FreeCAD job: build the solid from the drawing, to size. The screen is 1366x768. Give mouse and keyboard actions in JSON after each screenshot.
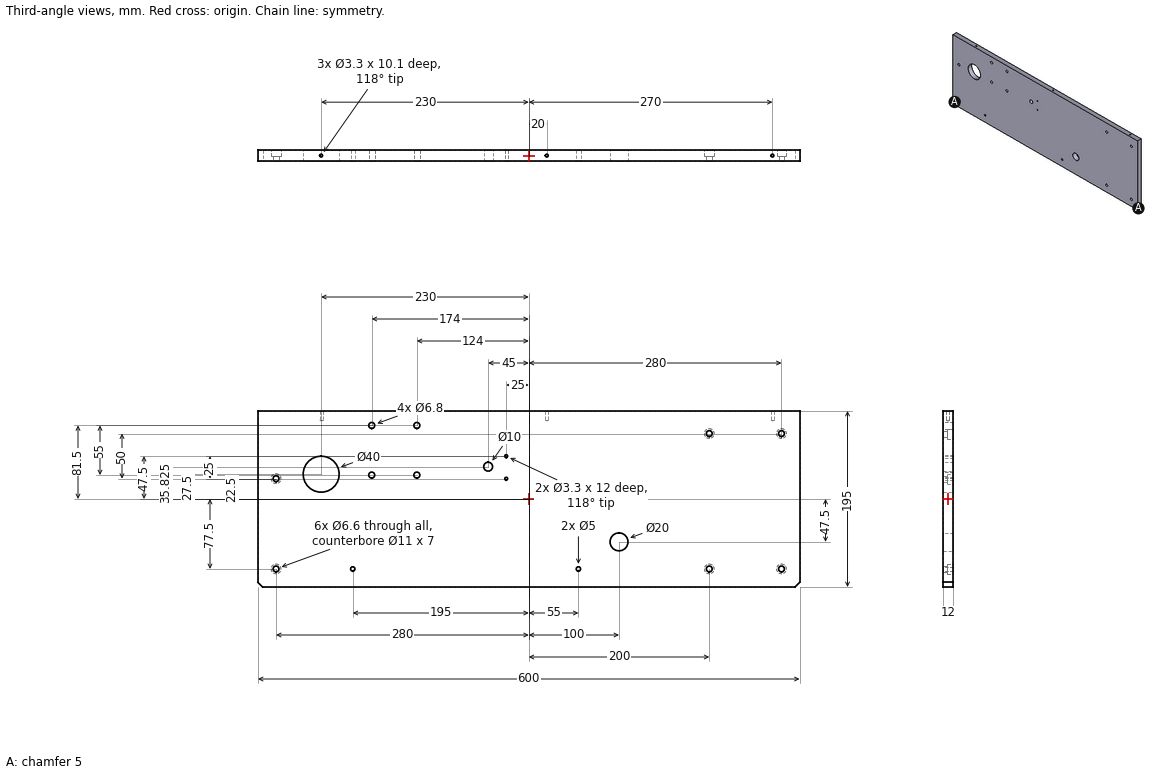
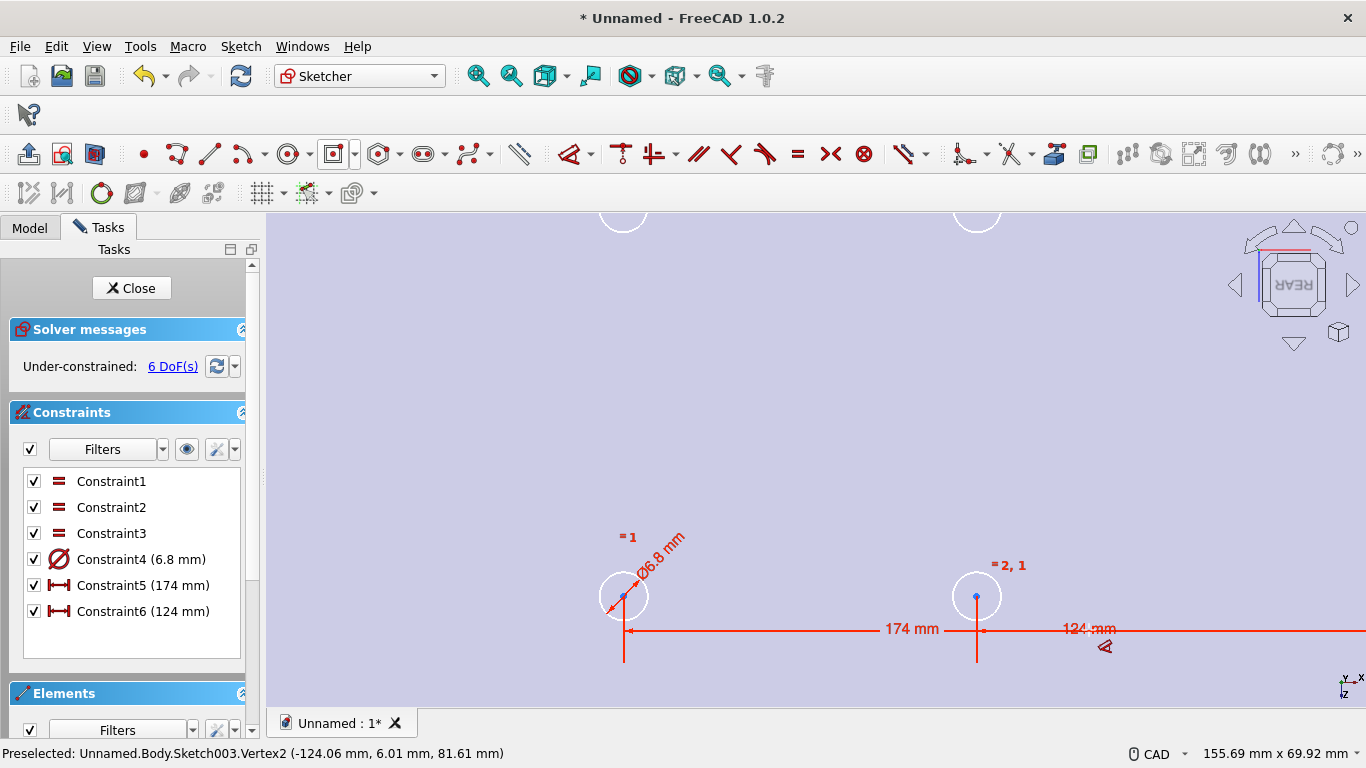
{"action": "scroll", "coordinate": [640, 579], "scroll_direction": "down", "scroll_amount": 2}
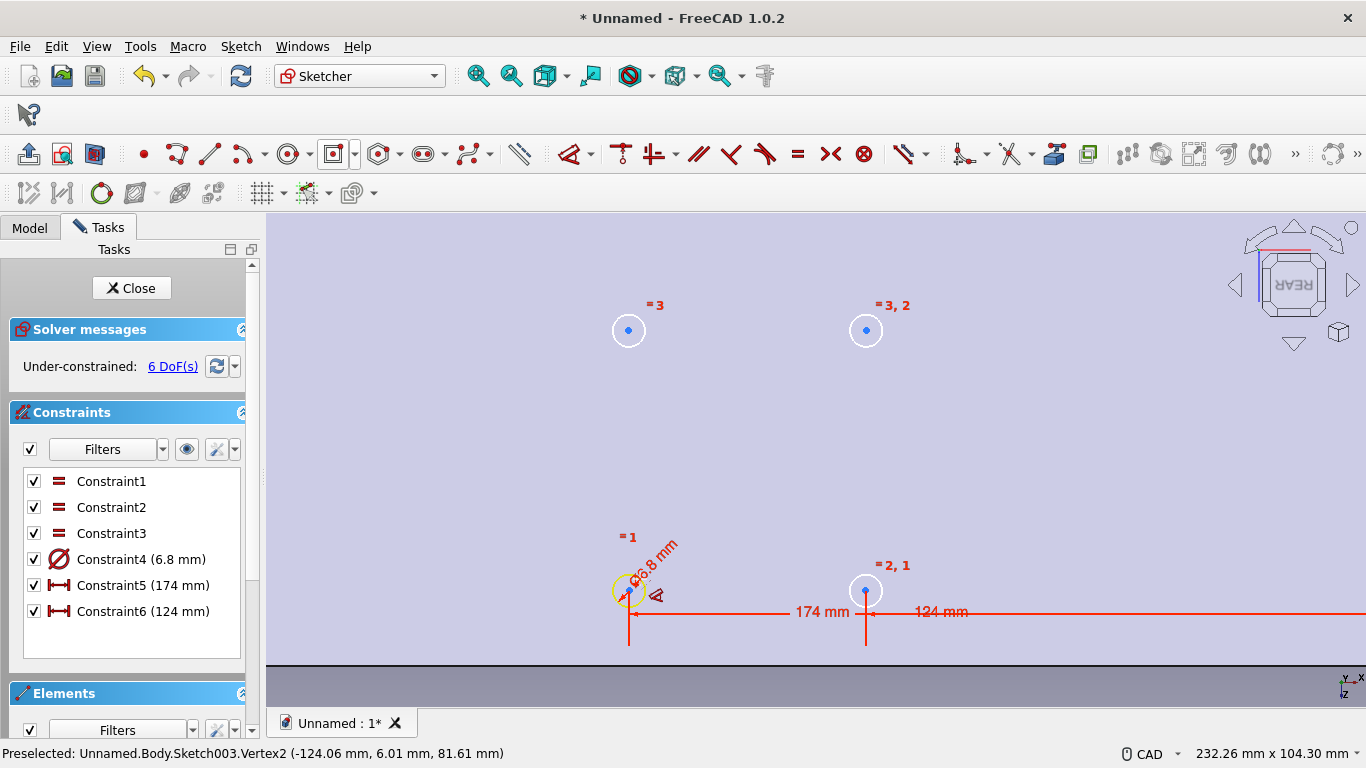
{"action": "left_click", "coordinate": [866, 331]}
{"action": "left_click", "coordinate": [1034, 365]}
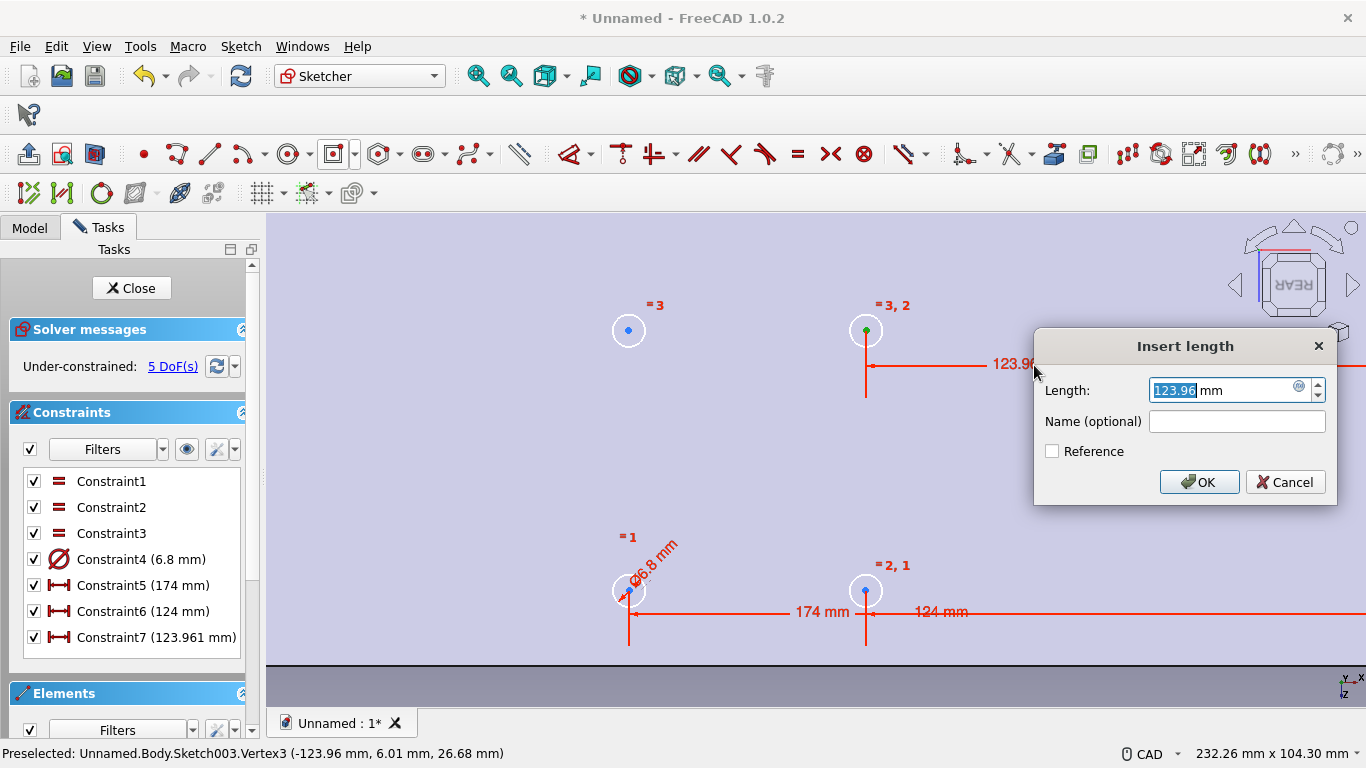
{"action": "type", "text": "124"}
{"action": "key", "text": "Return"}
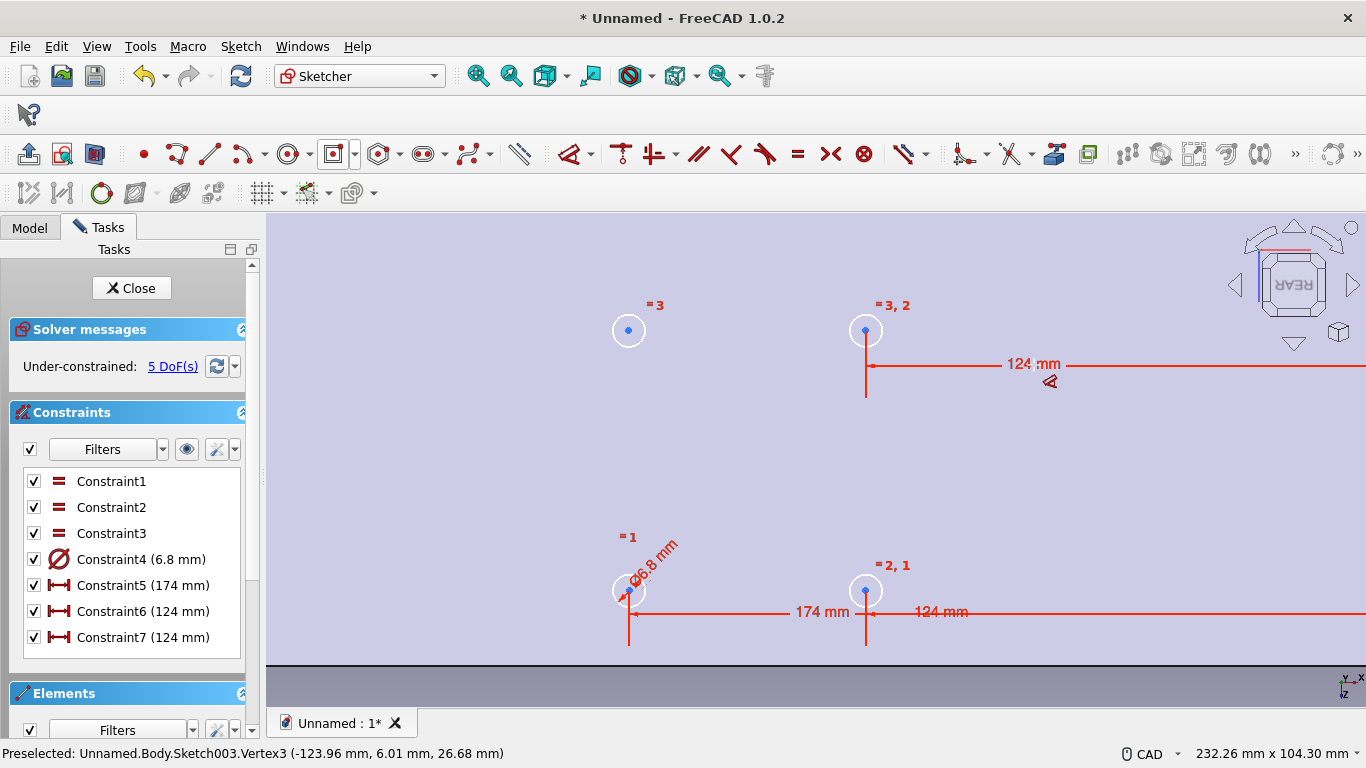
{"action": "left_click", "coordinate": [629, 331]}
{"action": "left_click", "coordinate": [915, 365]}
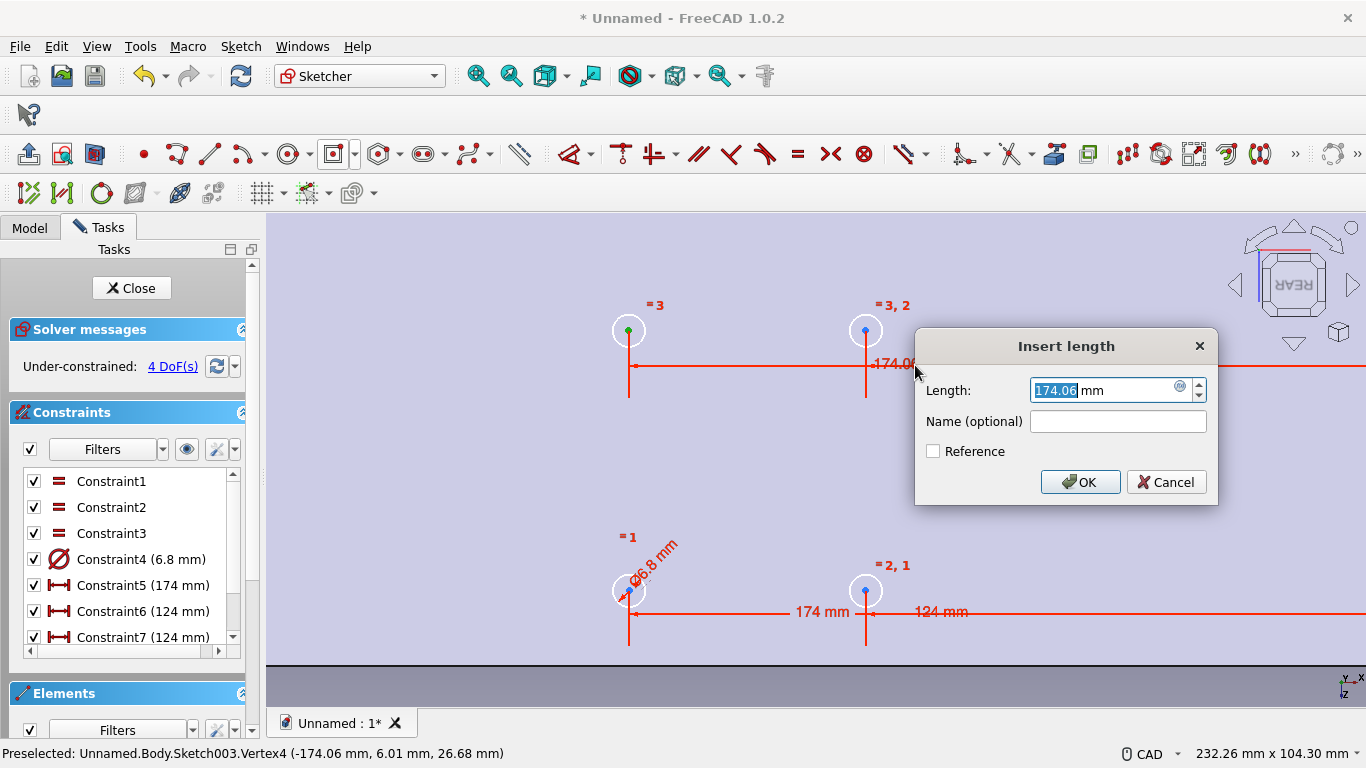
{"action": "type", "text": "174"}
{"action": "key", "text": "Return"}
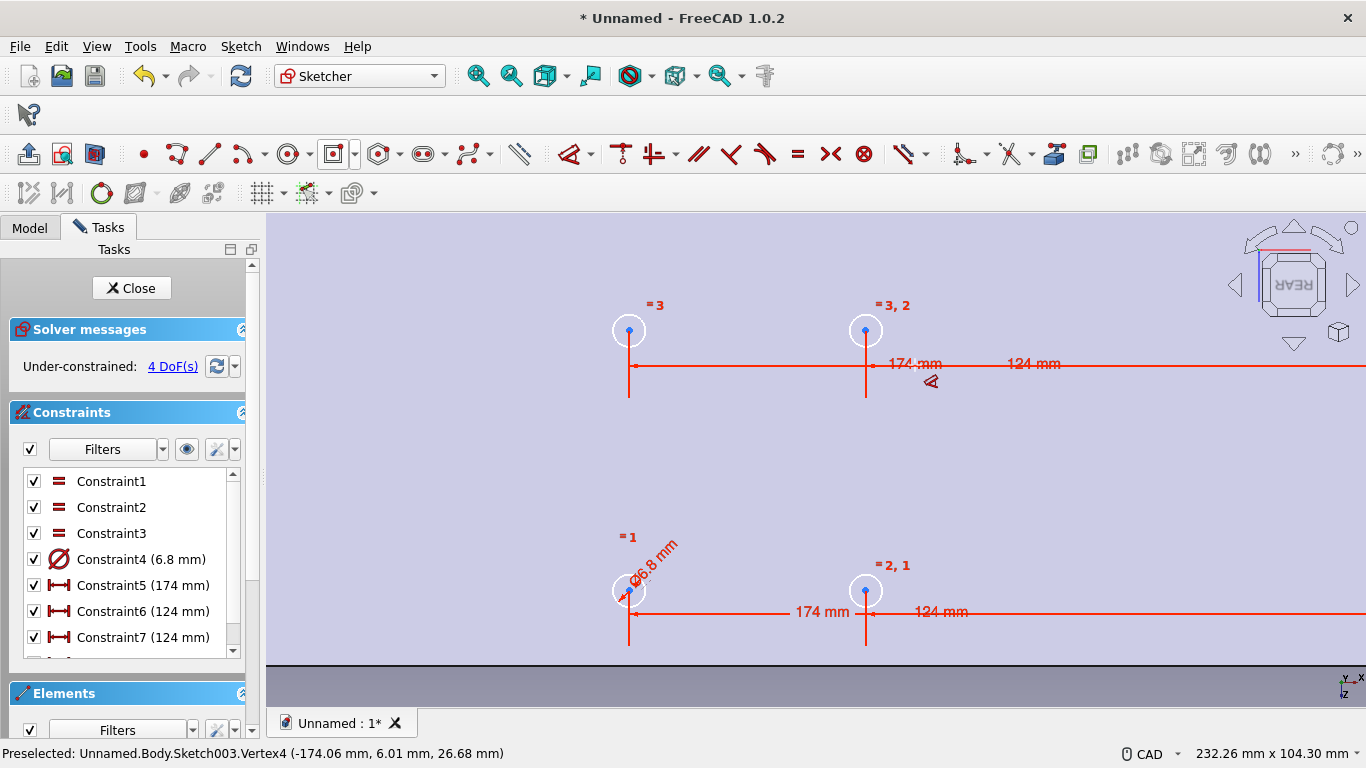
{"action": "left_click", "coordinate": [866, 591]}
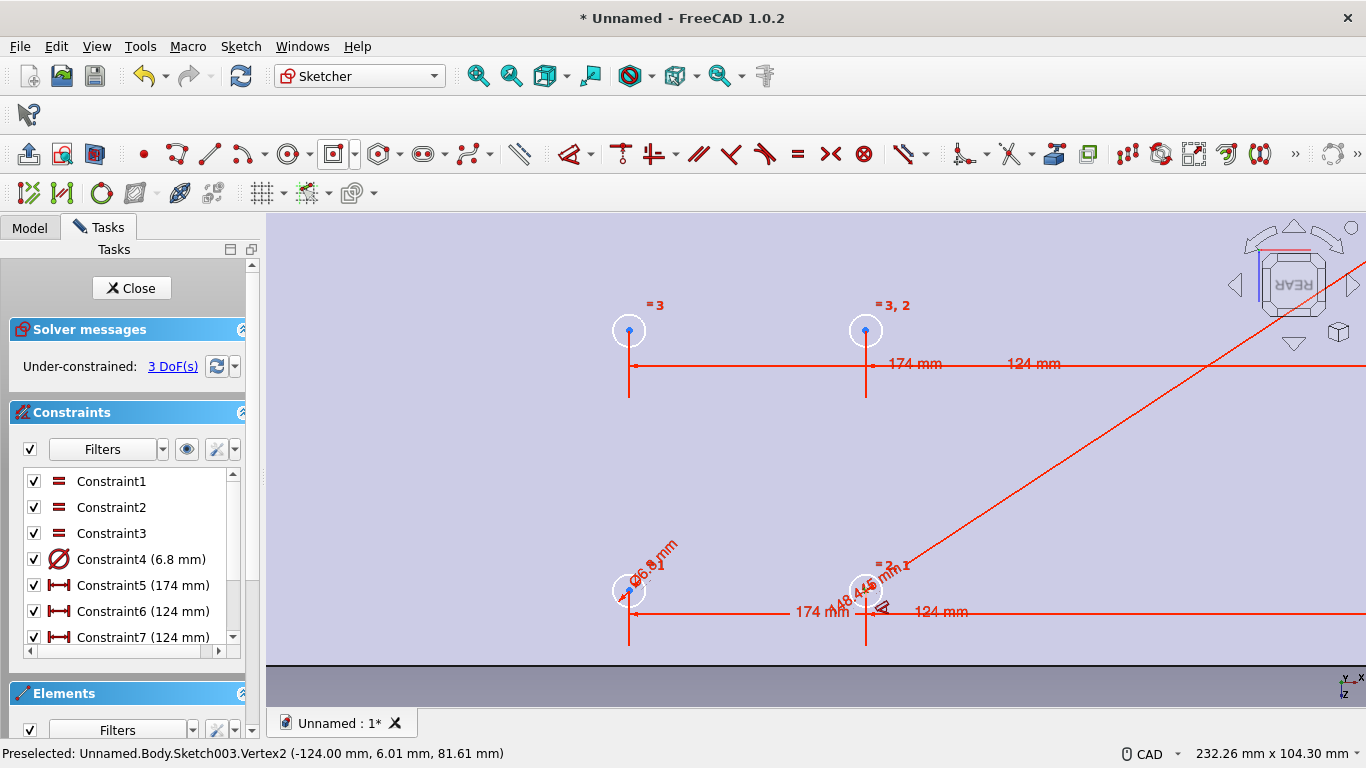
{"action": "left_click", "coordinate": [866, 331]}
{"action": "left_click", "coordinate": [900, 461]}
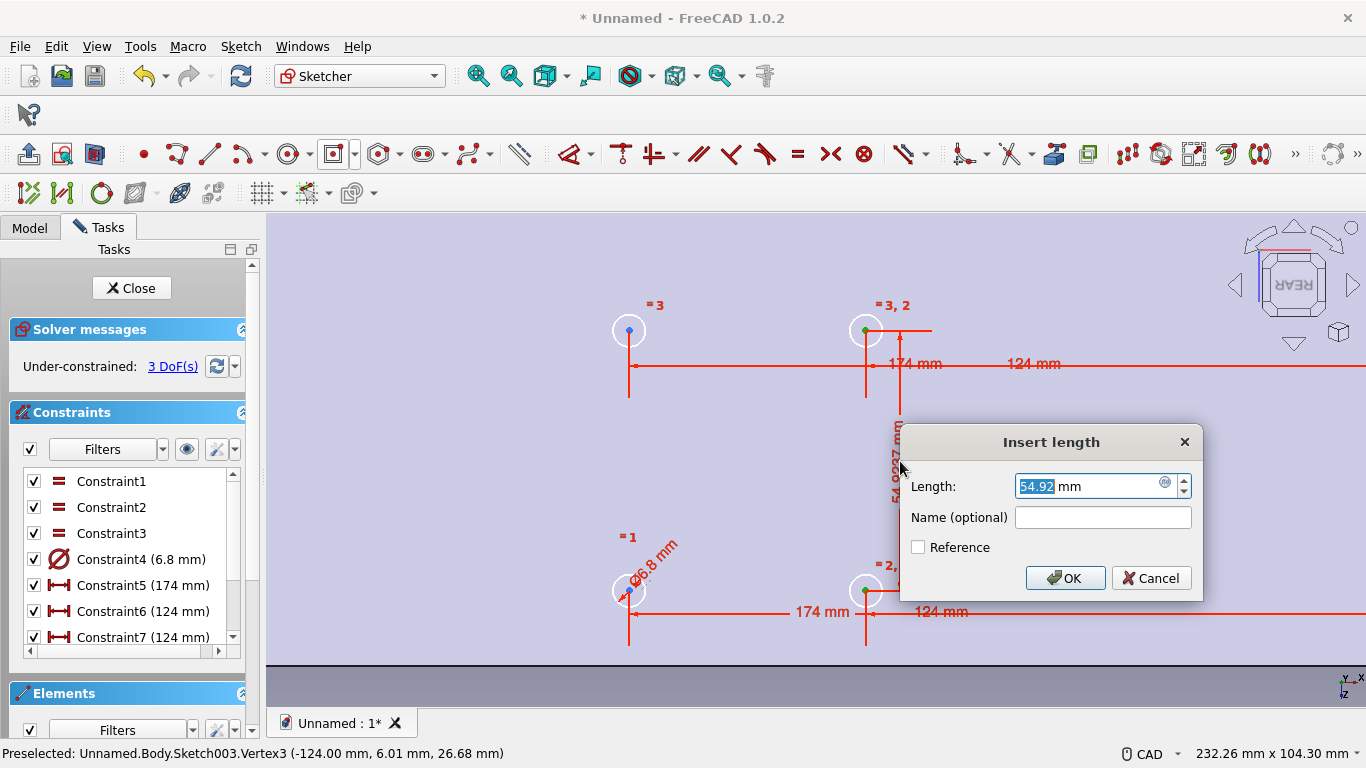
{"action": "type", "text": "55"}
{"action": "key", "text": "Return"}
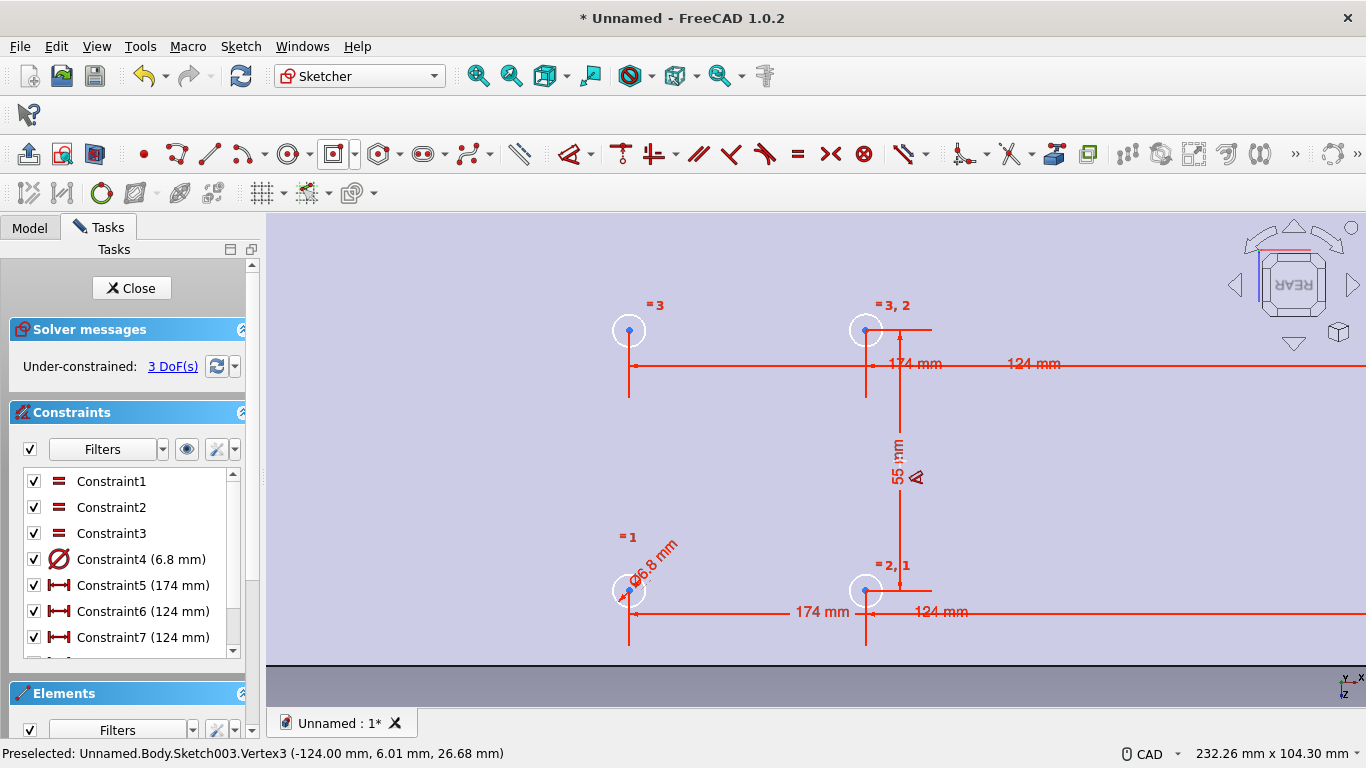
{"action": "left_click", "coordinate": [629, 591]}